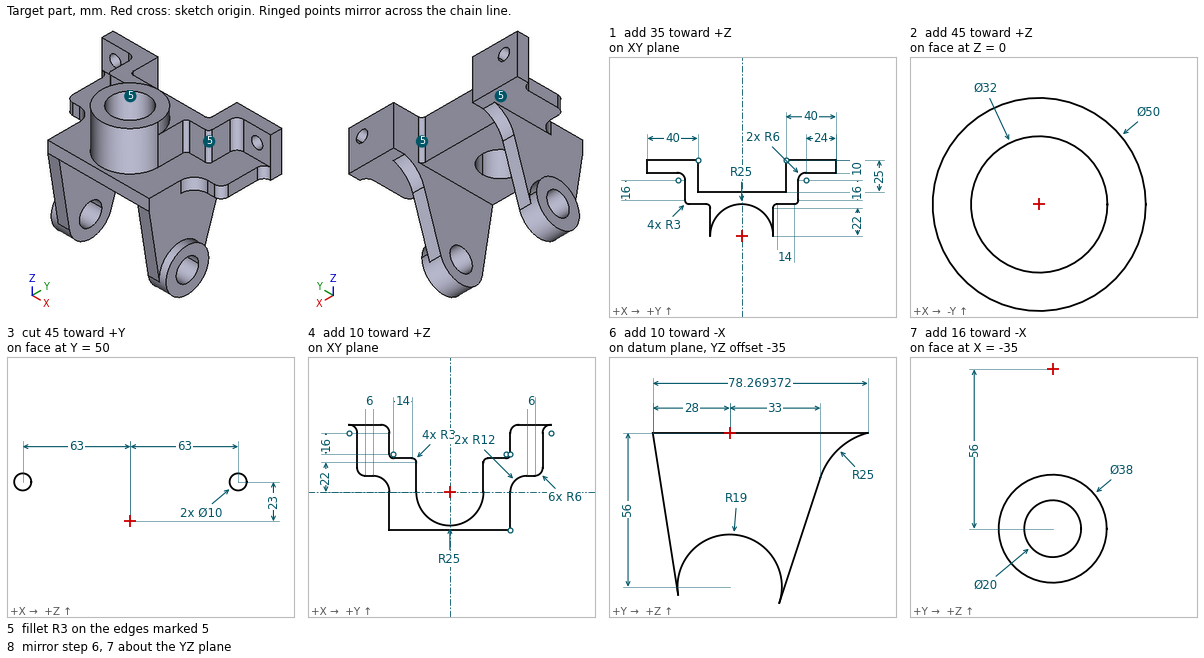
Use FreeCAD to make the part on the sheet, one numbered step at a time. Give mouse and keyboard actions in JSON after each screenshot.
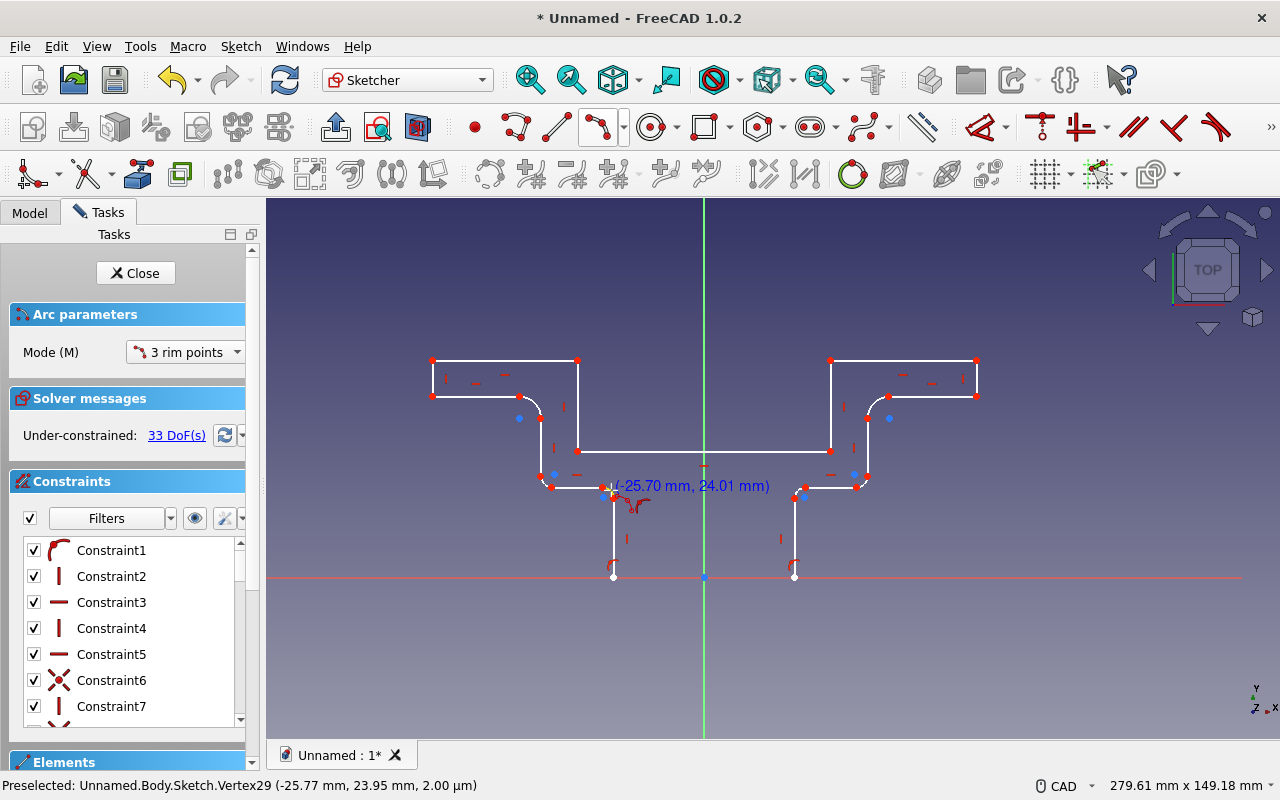
{"action": "left_click", "coordinate": [614, 578]}
{"action": "left_click", "coordinate": [795, 578]}
{"action": "left_click", "coordinate": [732, 491]}
{"action": "key", "text": "Escape"}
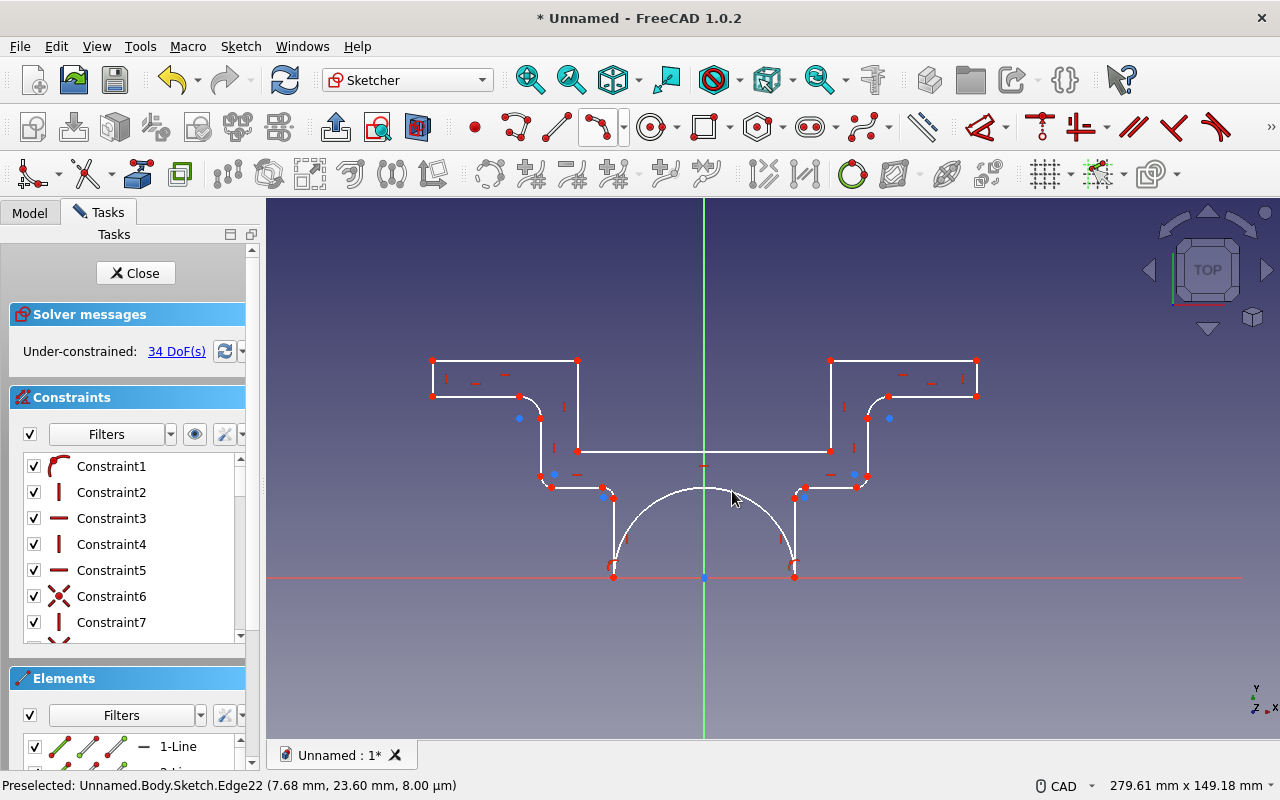
{"action": "left_click", "coordinate": [795, 523]}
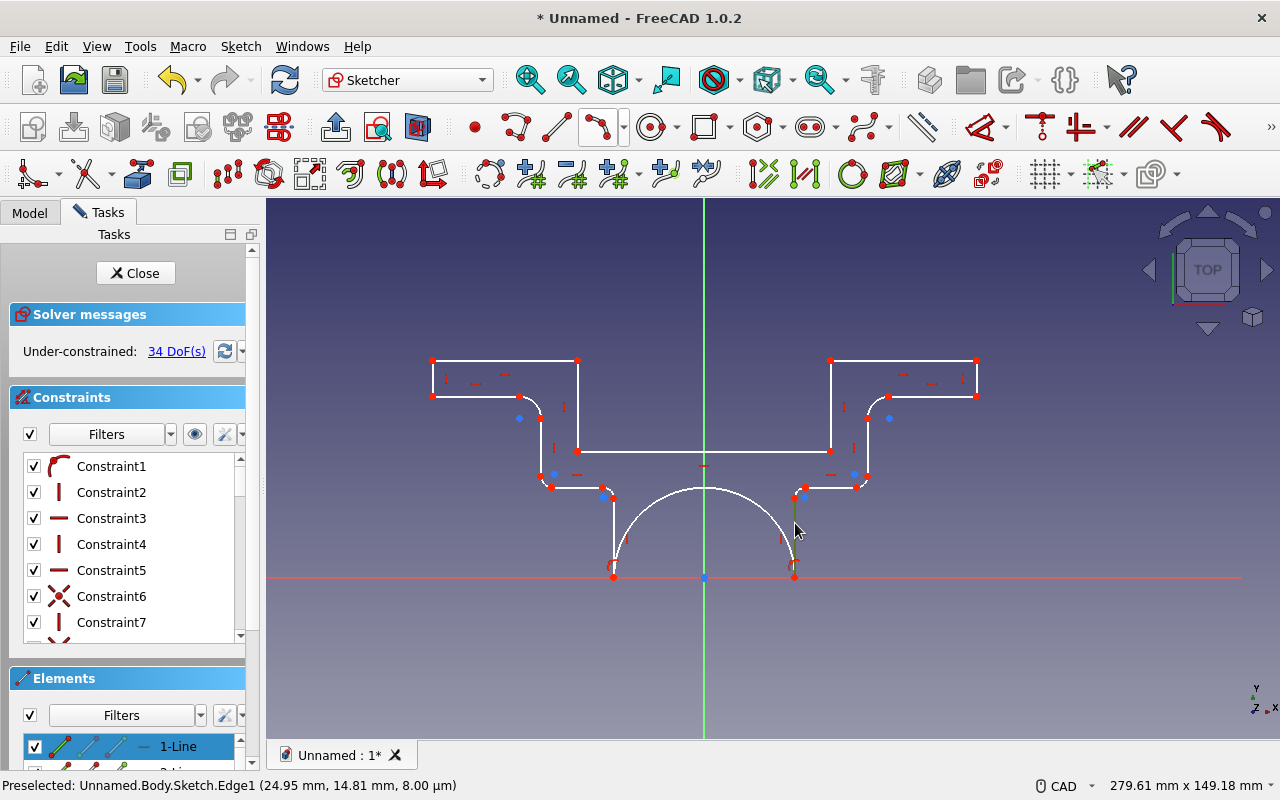
{"action": "scroll", "coordinate": [798, 491], "scroll_direction": "up", "scroll_amount": 3}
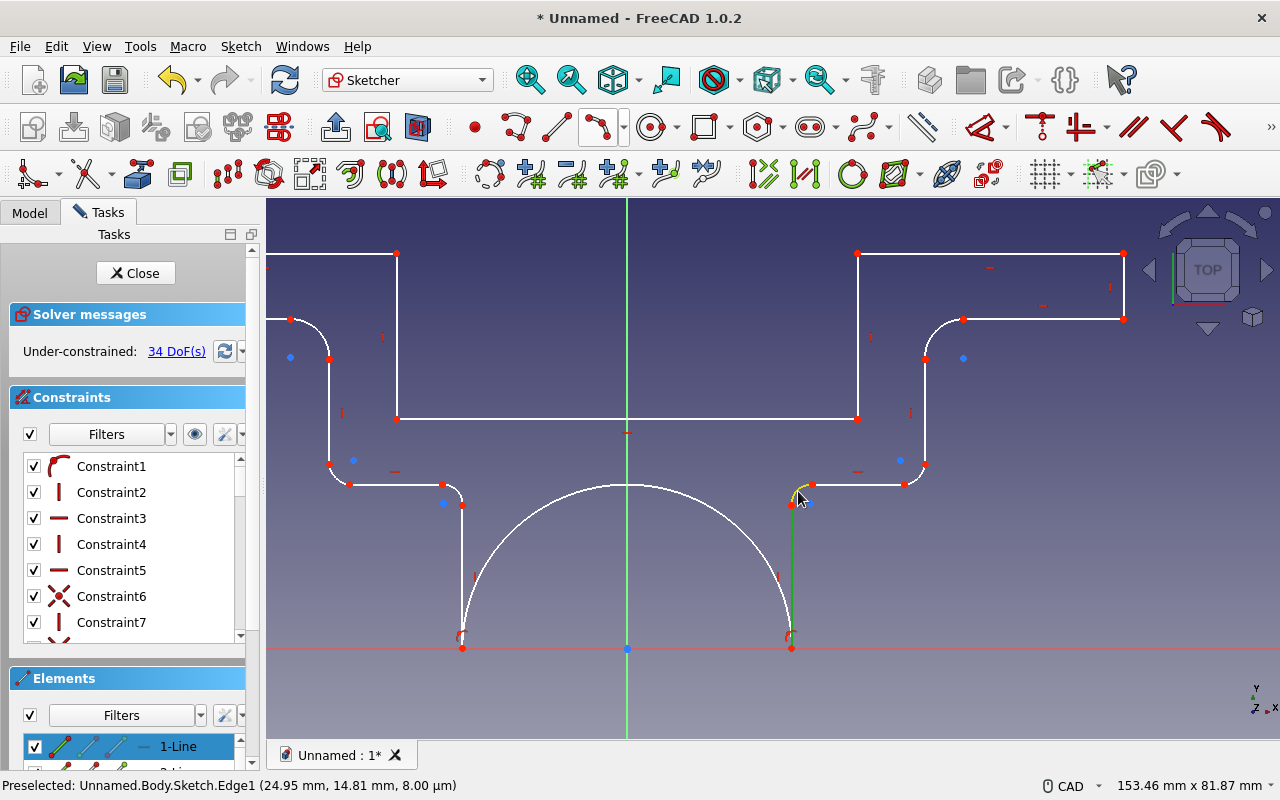
{"action": "left_click", "coordinate": [797, 490]}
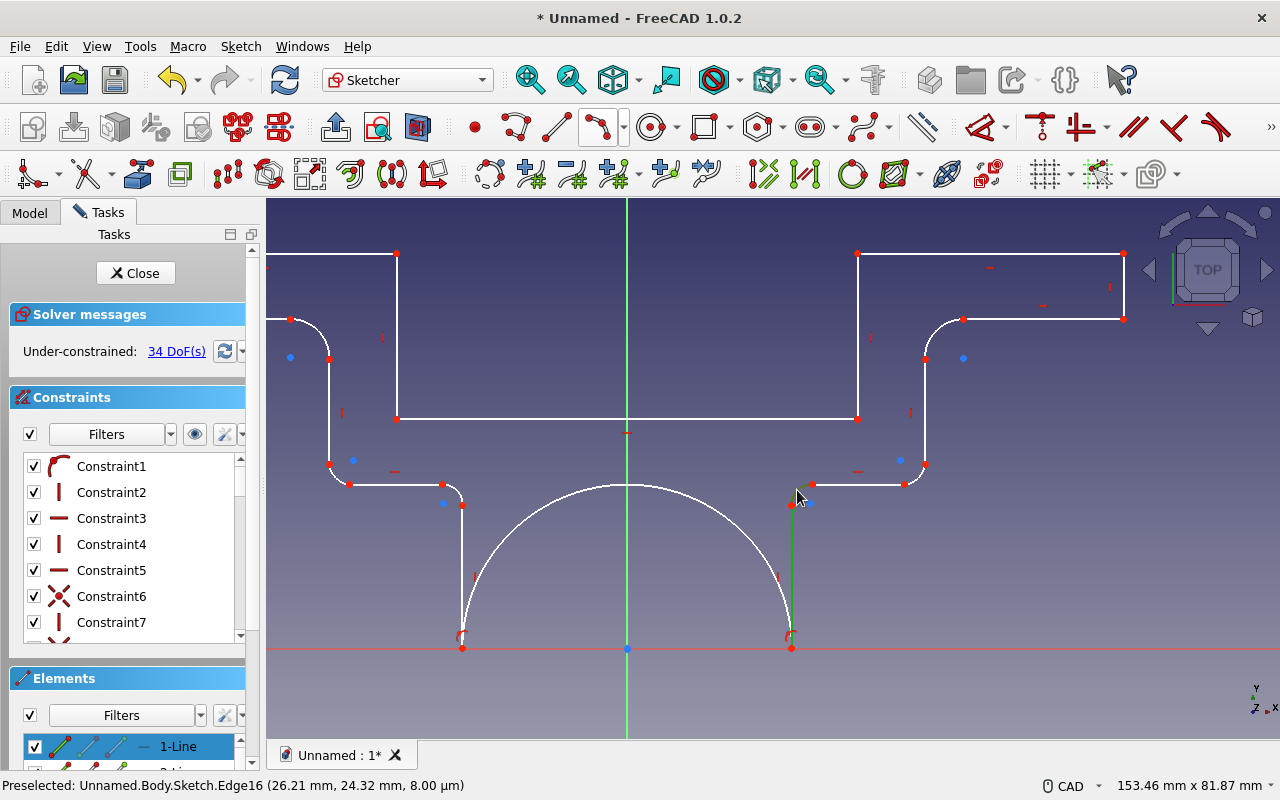
{"action": "left_click", "coordinate": [1216, 128]}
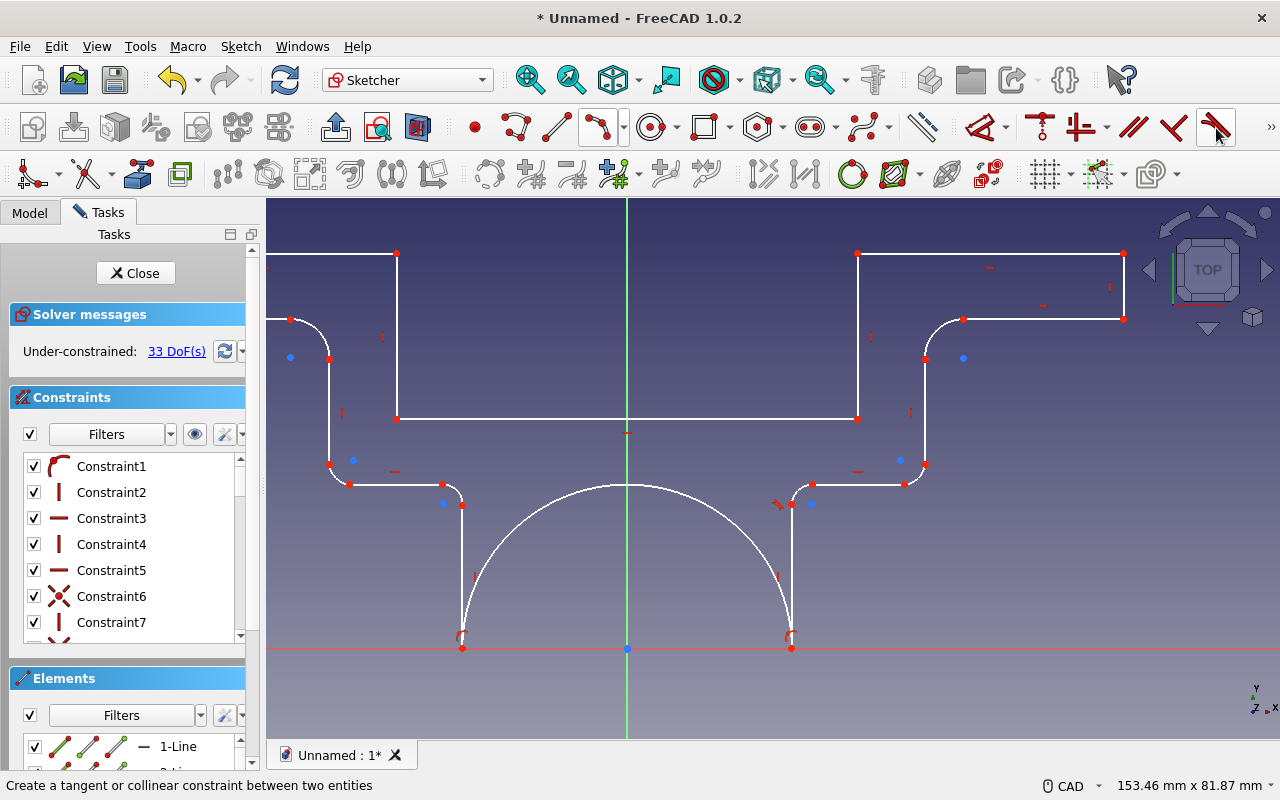
{"action": "left_click", "coordinate": [792, 548]}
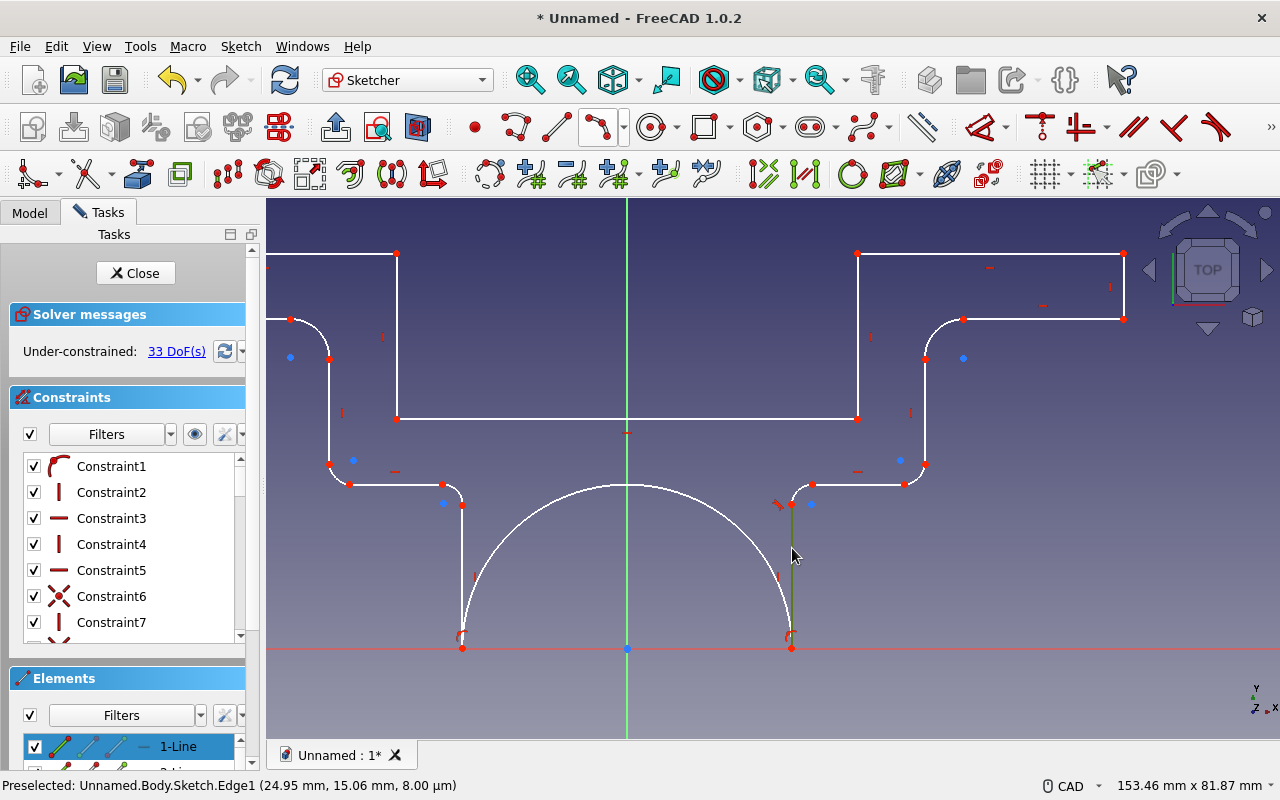
{"action": "left_click", "coordinate": [724, 516]}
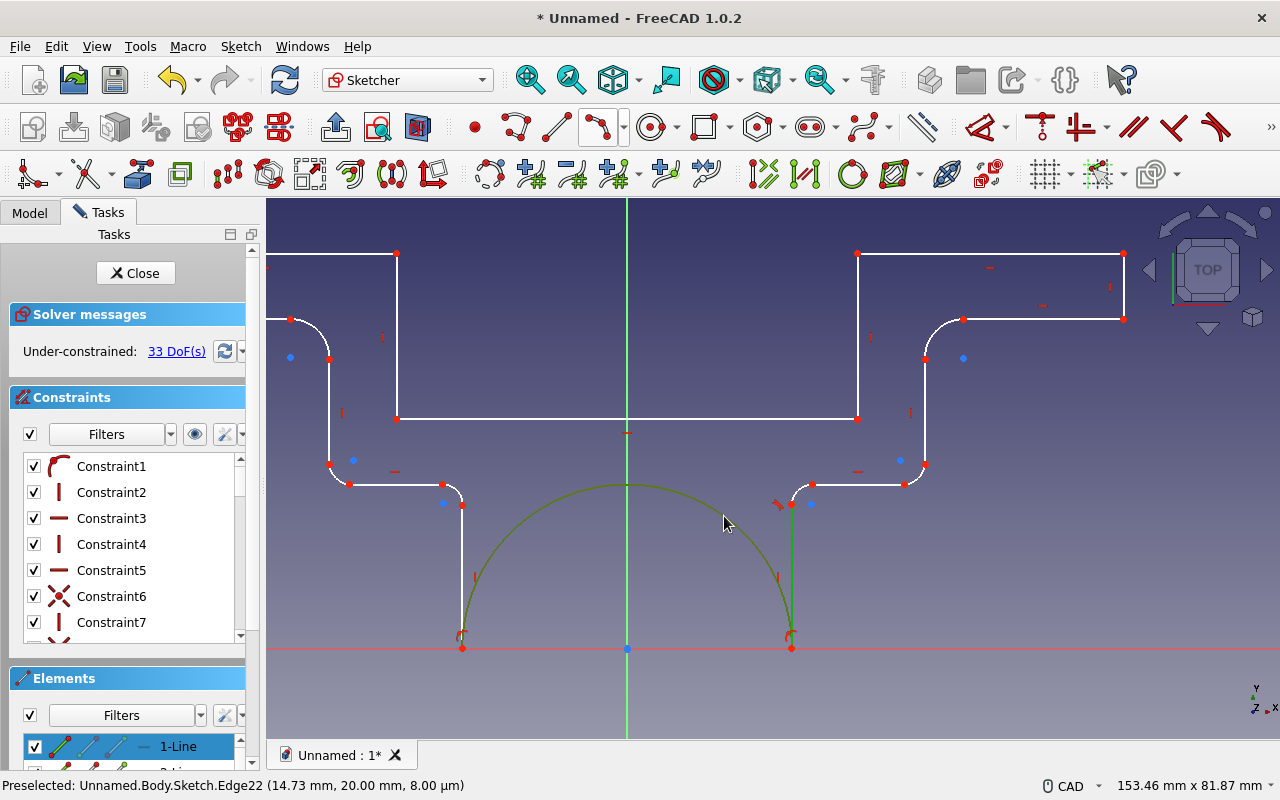
{"action": "left_click", "coordinate": [1216, 128]}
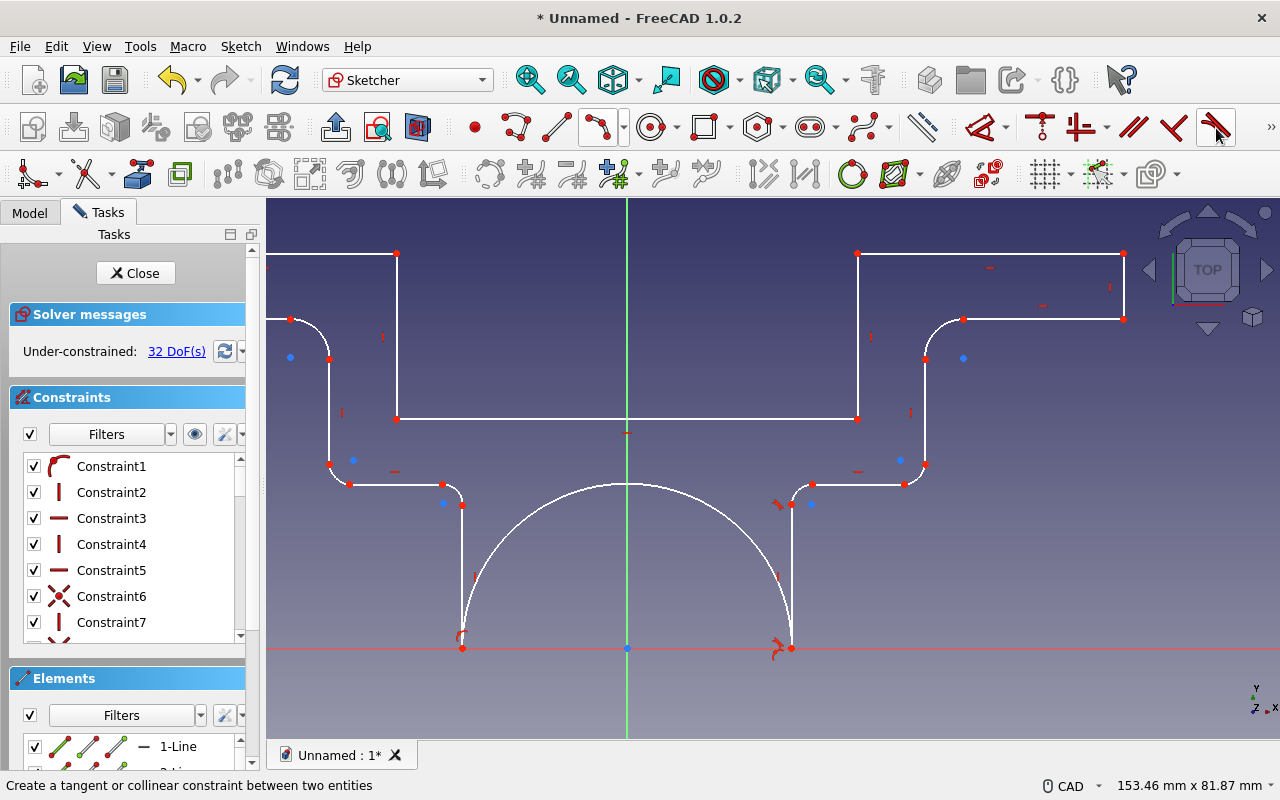
{"action": "left_click", "coordinate": [840, 485]}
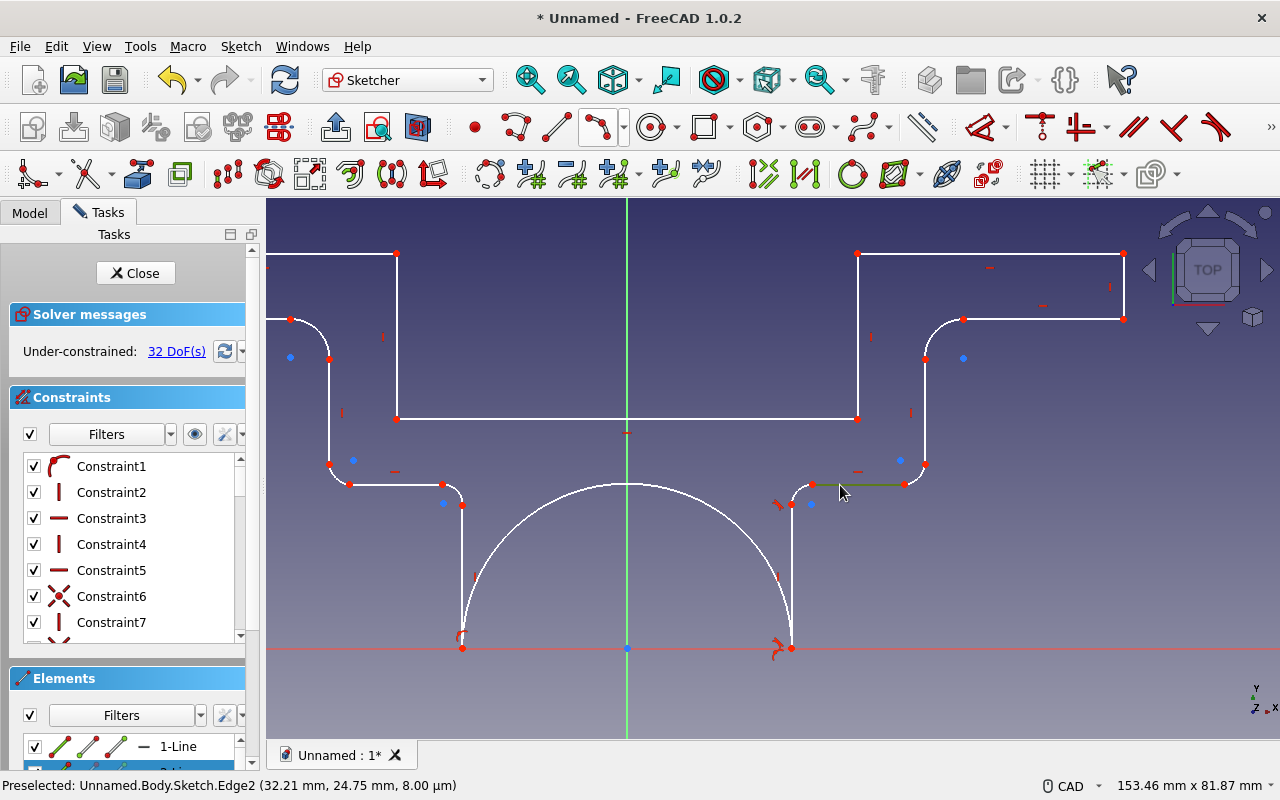
{"action": "scroll", "coordinate": [803, 487], "scroll_direction": "up", "scroll_amount": 2}